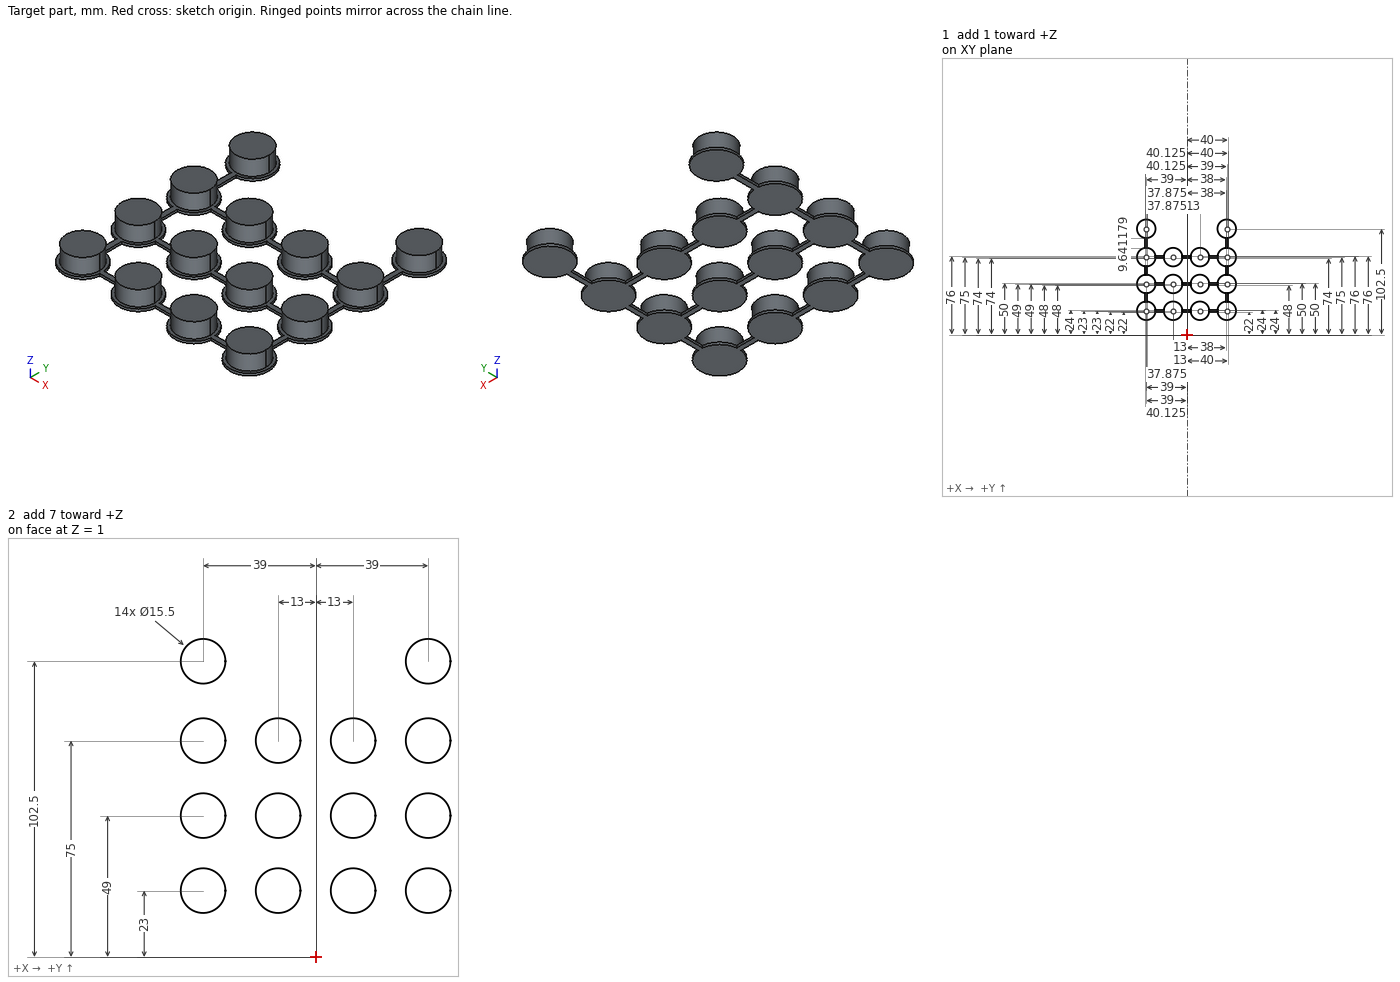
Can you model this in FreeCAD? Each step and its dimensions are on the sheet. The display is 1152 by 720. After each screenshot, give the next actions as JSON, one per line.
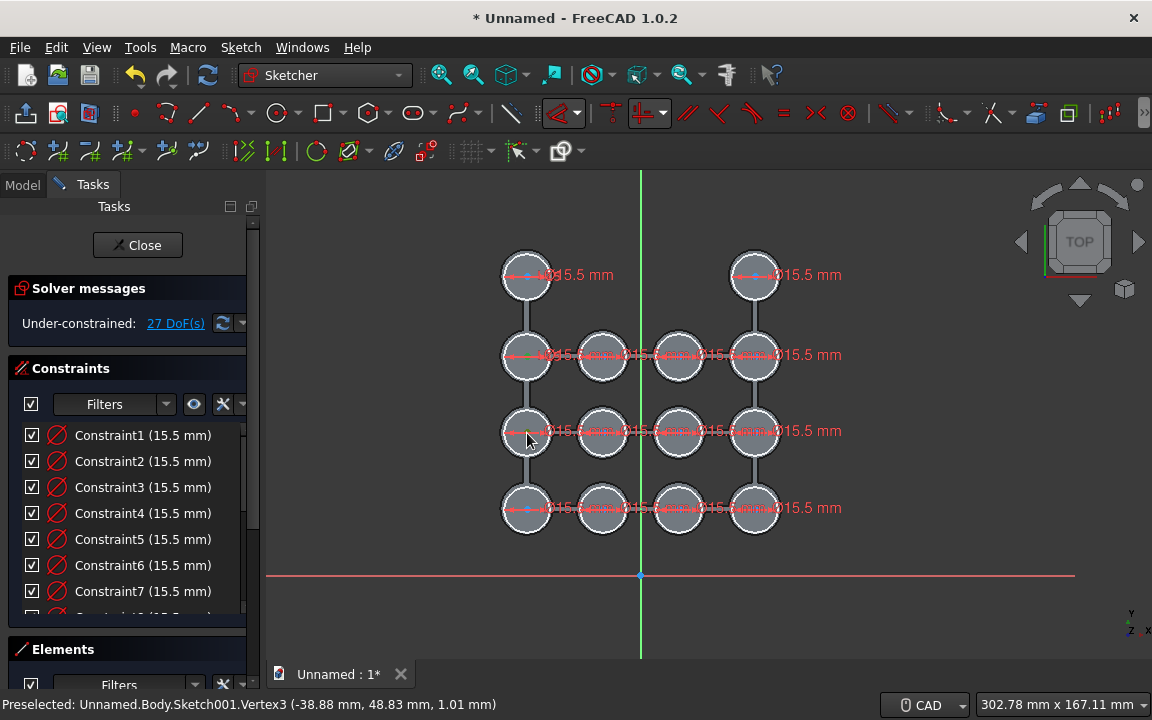
{"action": "key", "text": "v"}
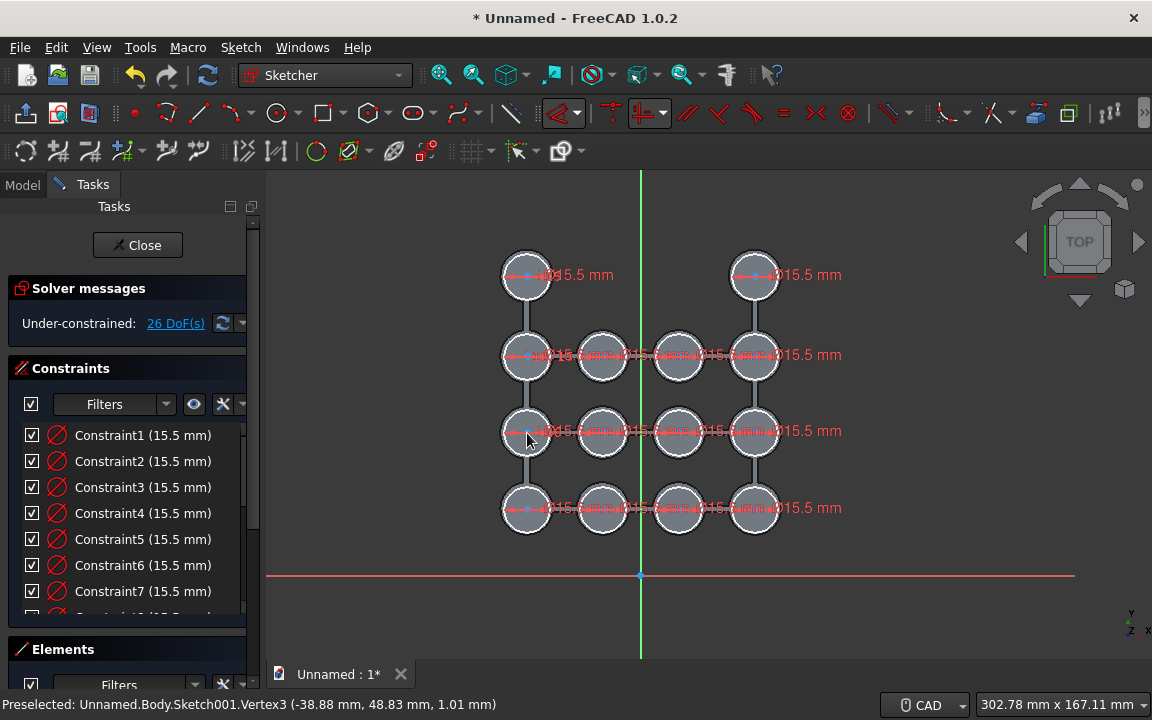
{"action": "left_click", "coordinate": [527, 433]}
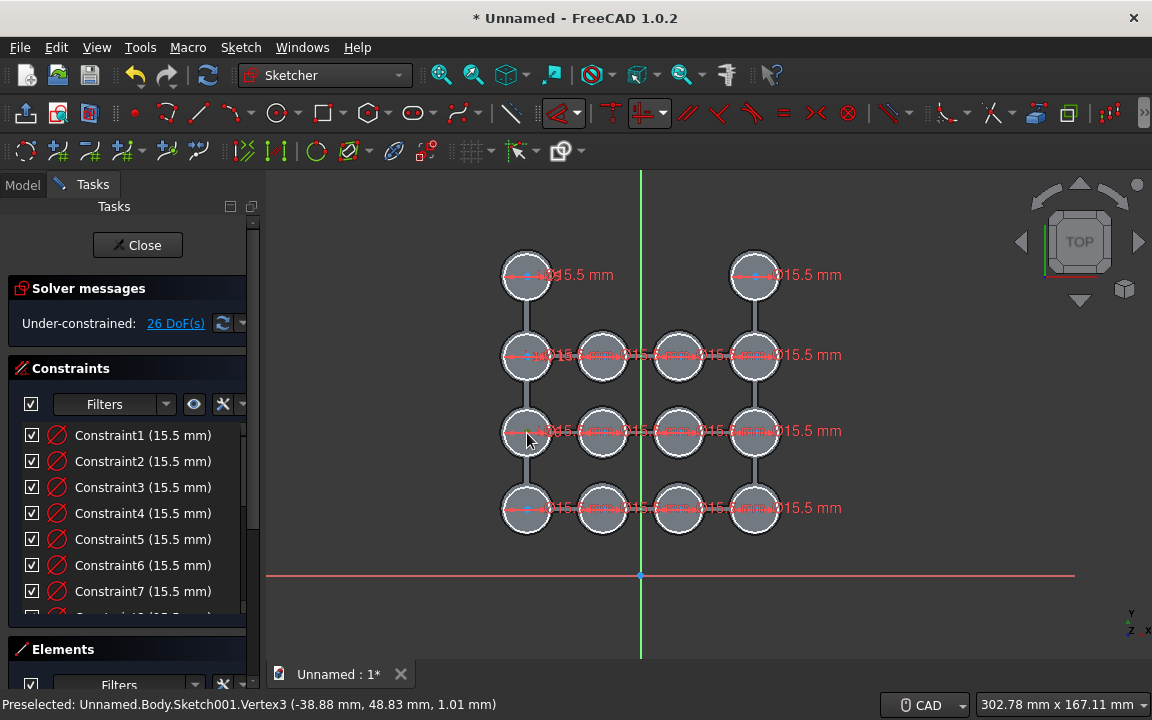
{"action": "left_click", "coordinate": [527, 510]}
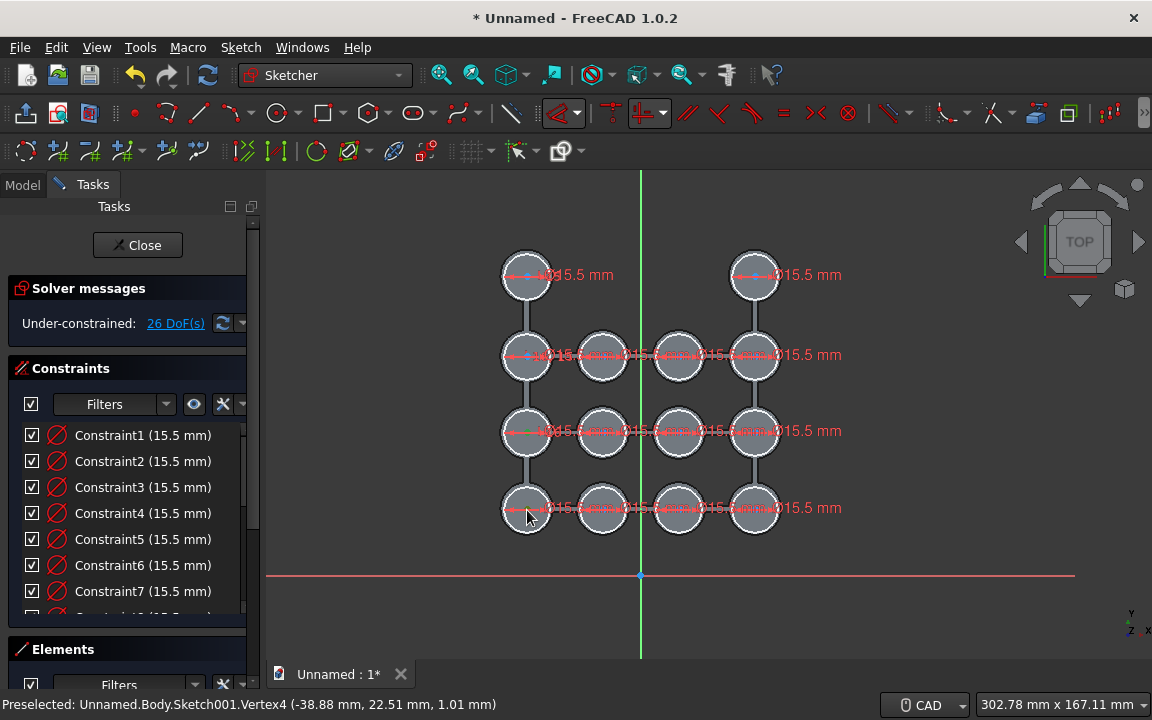
{"action": "left_click", "coordinate": [666, 114]}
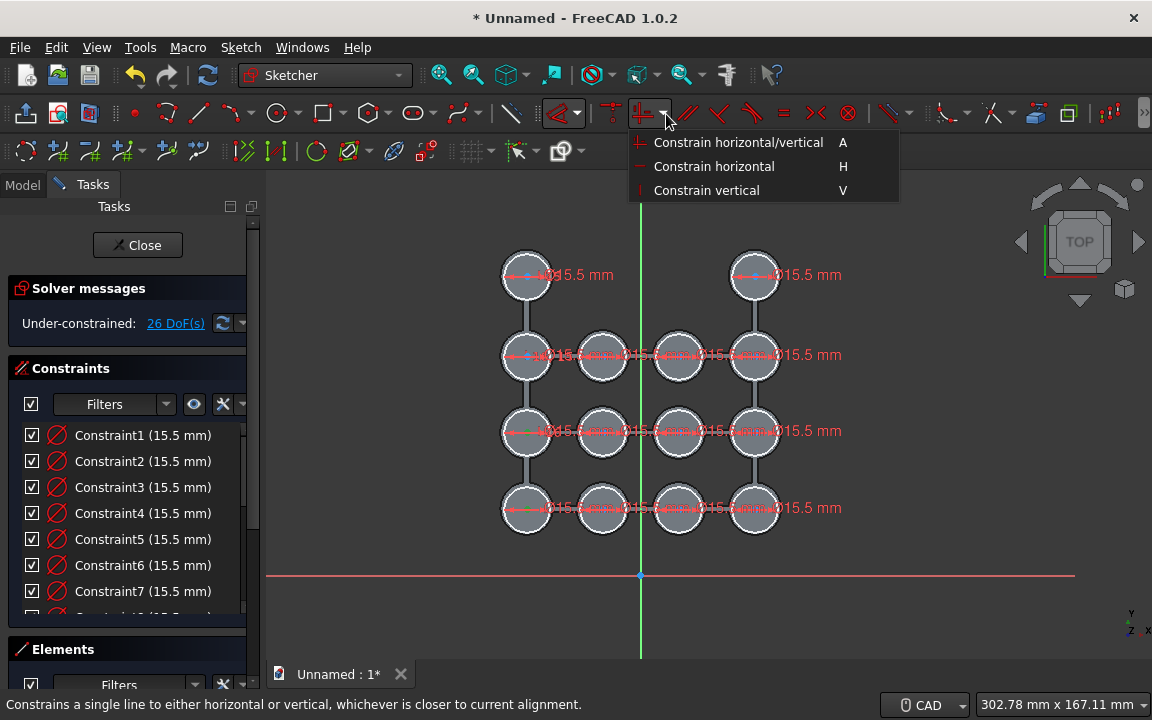
{"action": "left_click", "coordinate": [764, 190]}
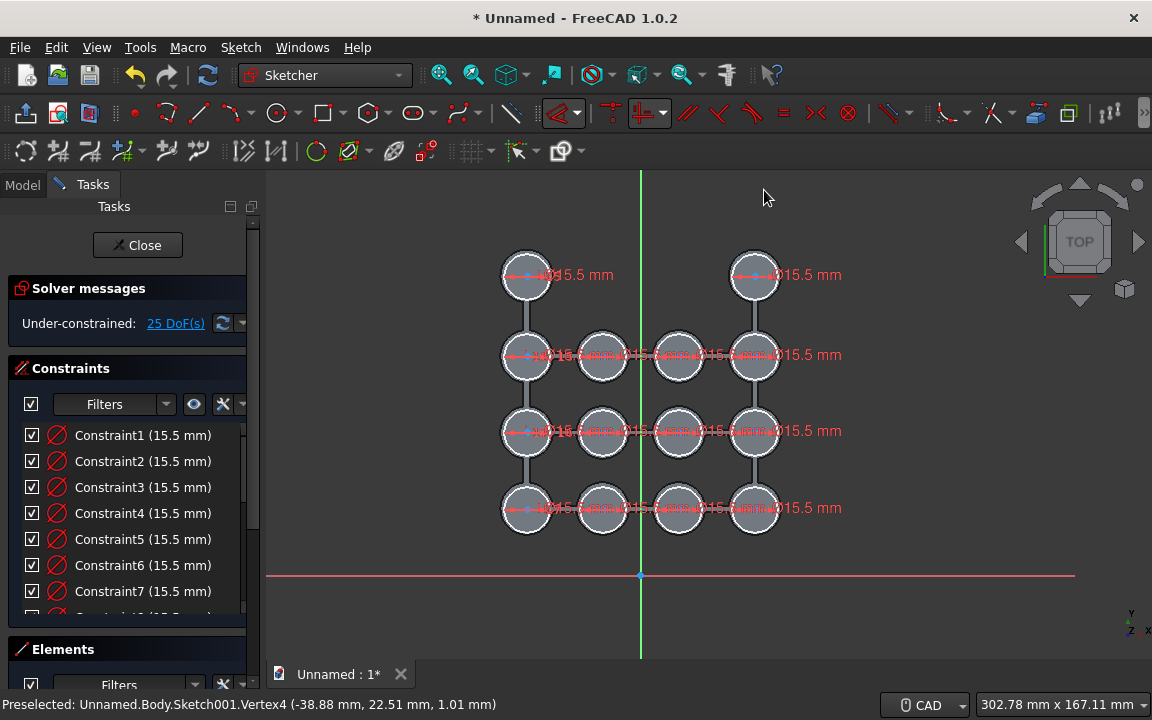
{"action": "left_click", "coordinate": [527, 357]}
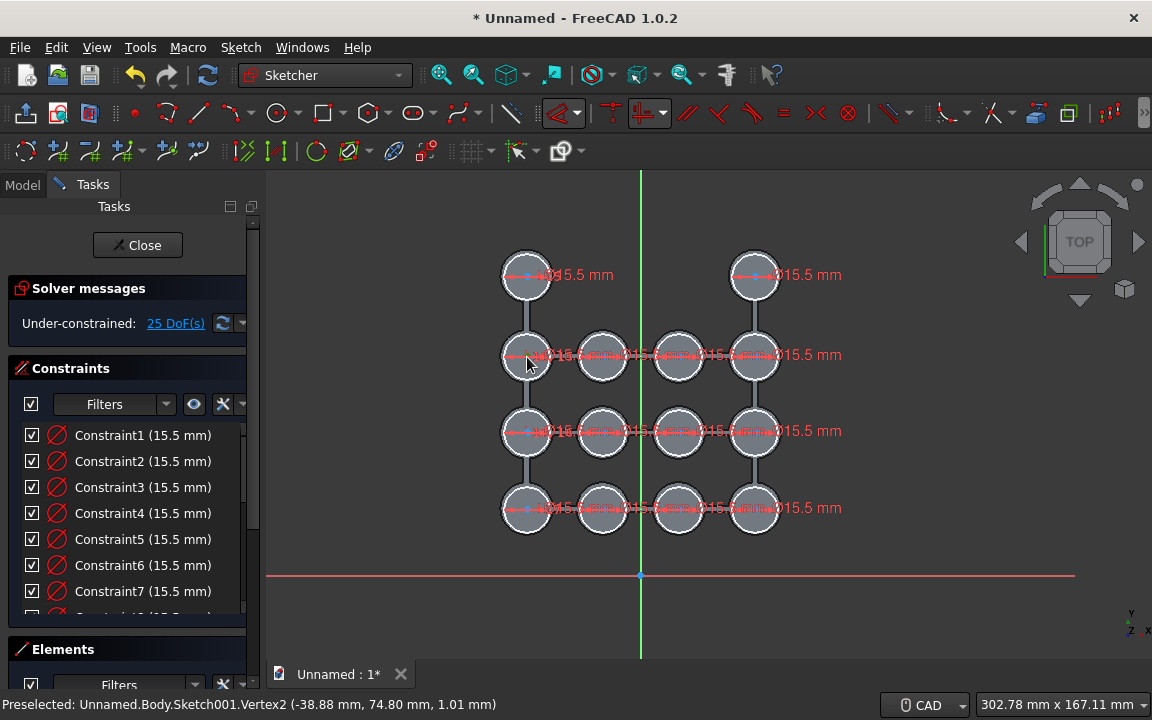
{"action": "left_click", "coordinate": [603, 357]}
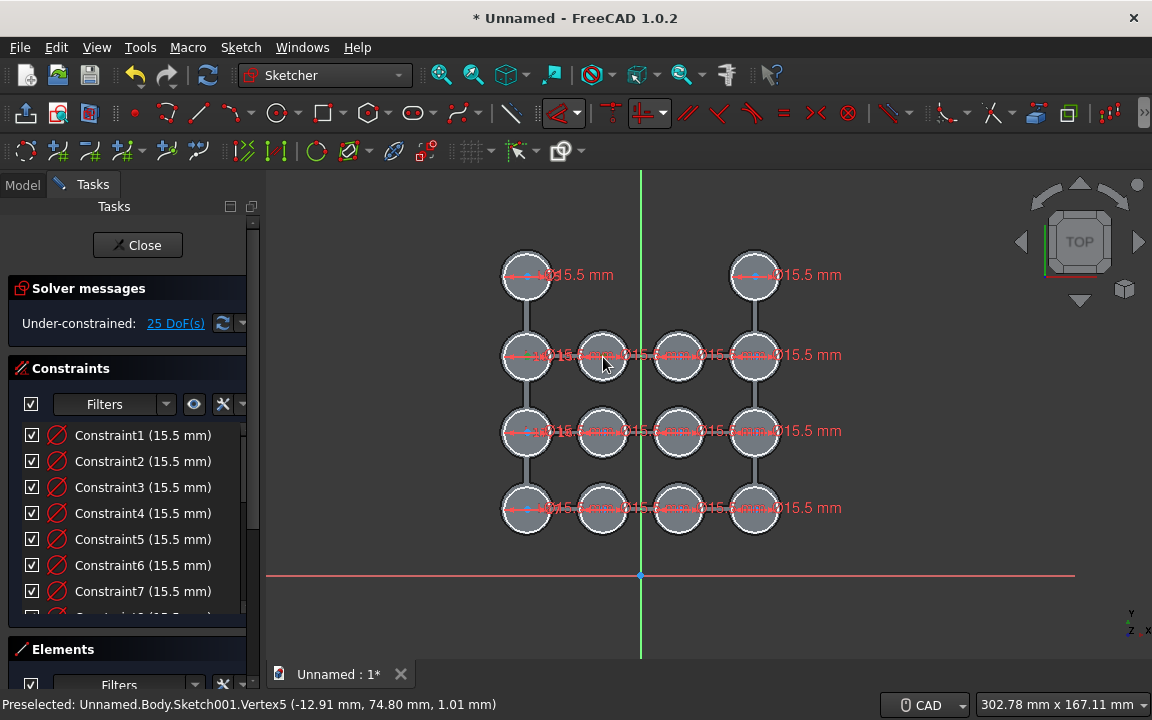
{"action": "key", "text": "h"}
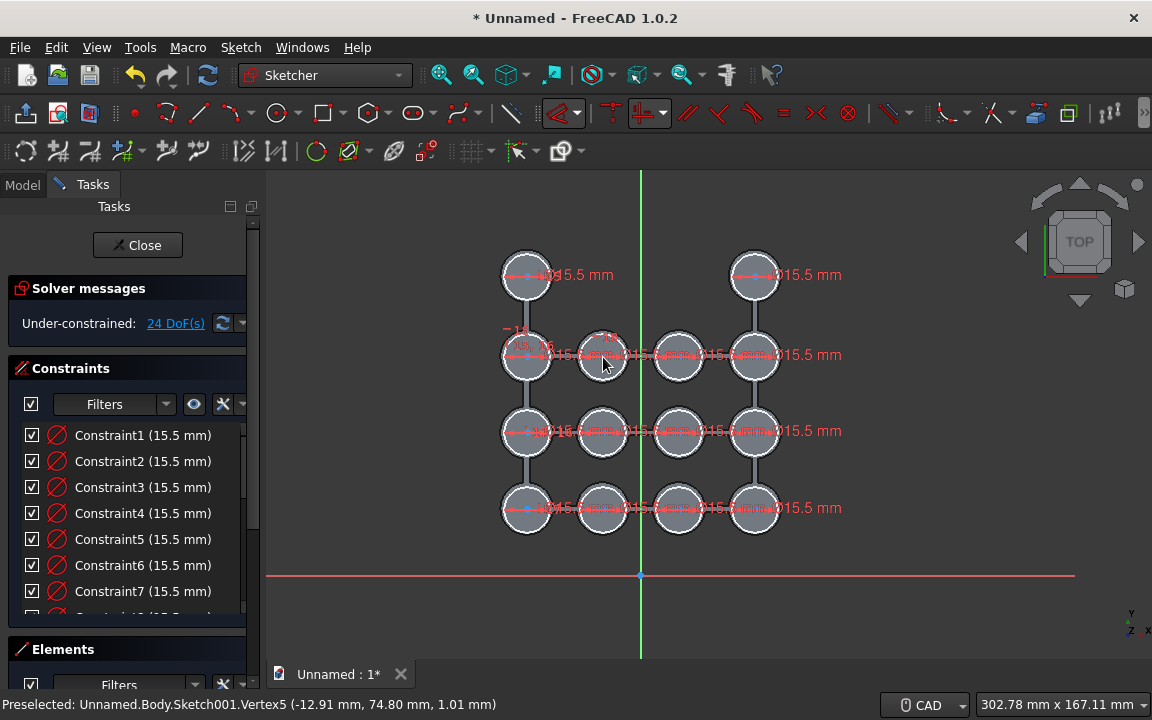
{"action": "left_click", "coordinate": [603, 357]}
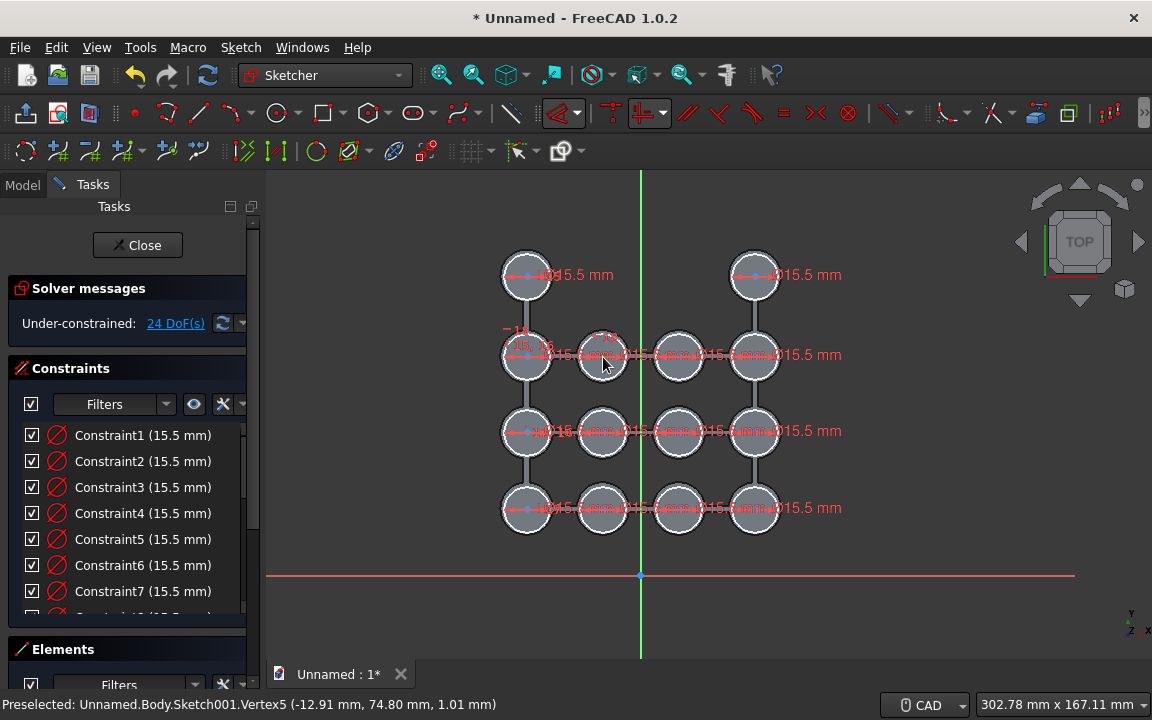
{"action": "left_click", "coordinate": [603, 433]}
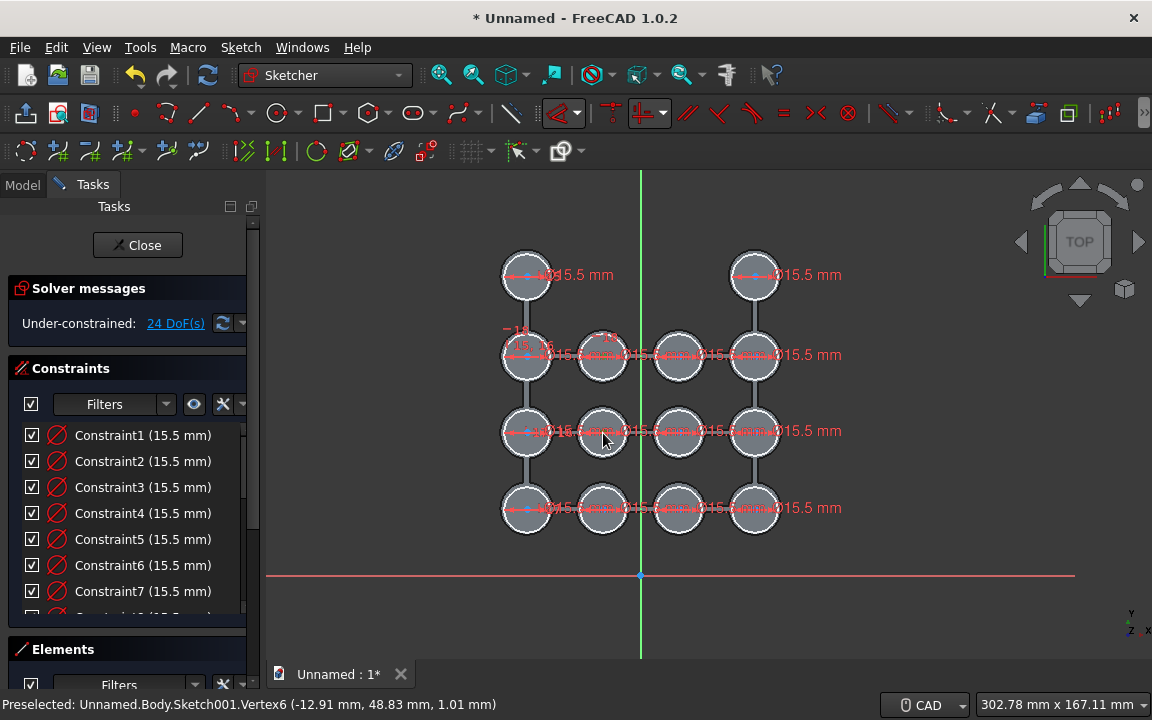
{"action": "key", "text": "v"}